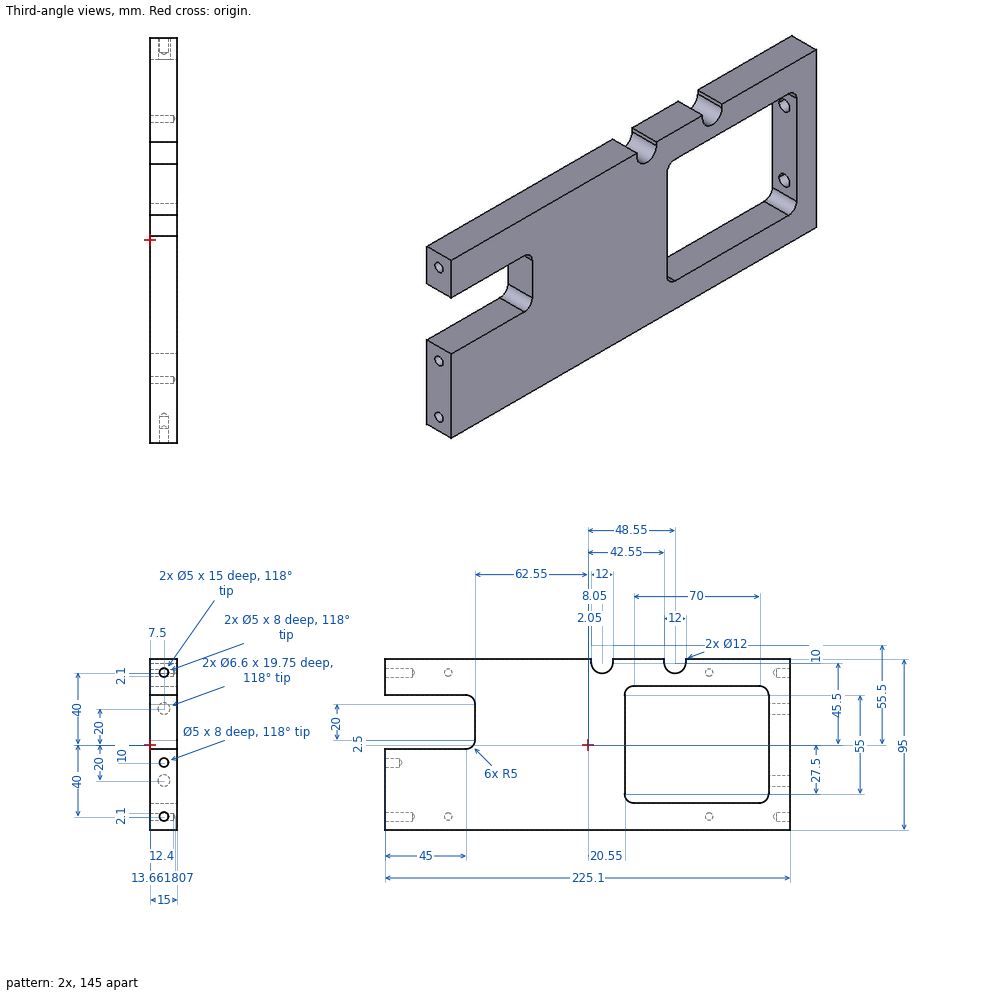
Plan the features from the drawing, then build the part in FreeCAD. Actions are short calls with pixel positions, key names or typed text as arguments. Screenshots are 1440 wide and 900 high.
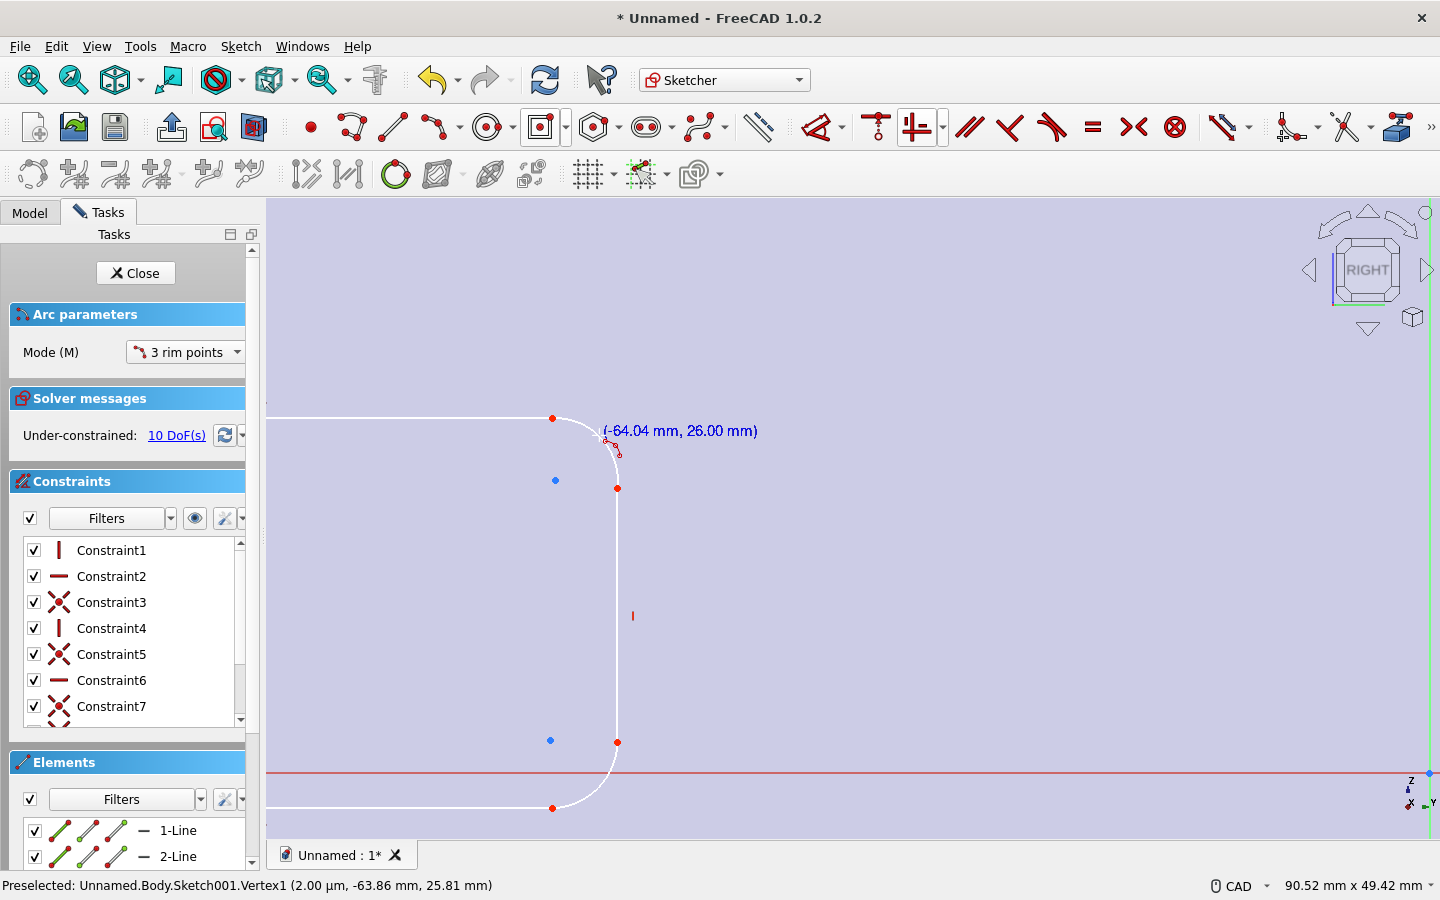
click(393, 128)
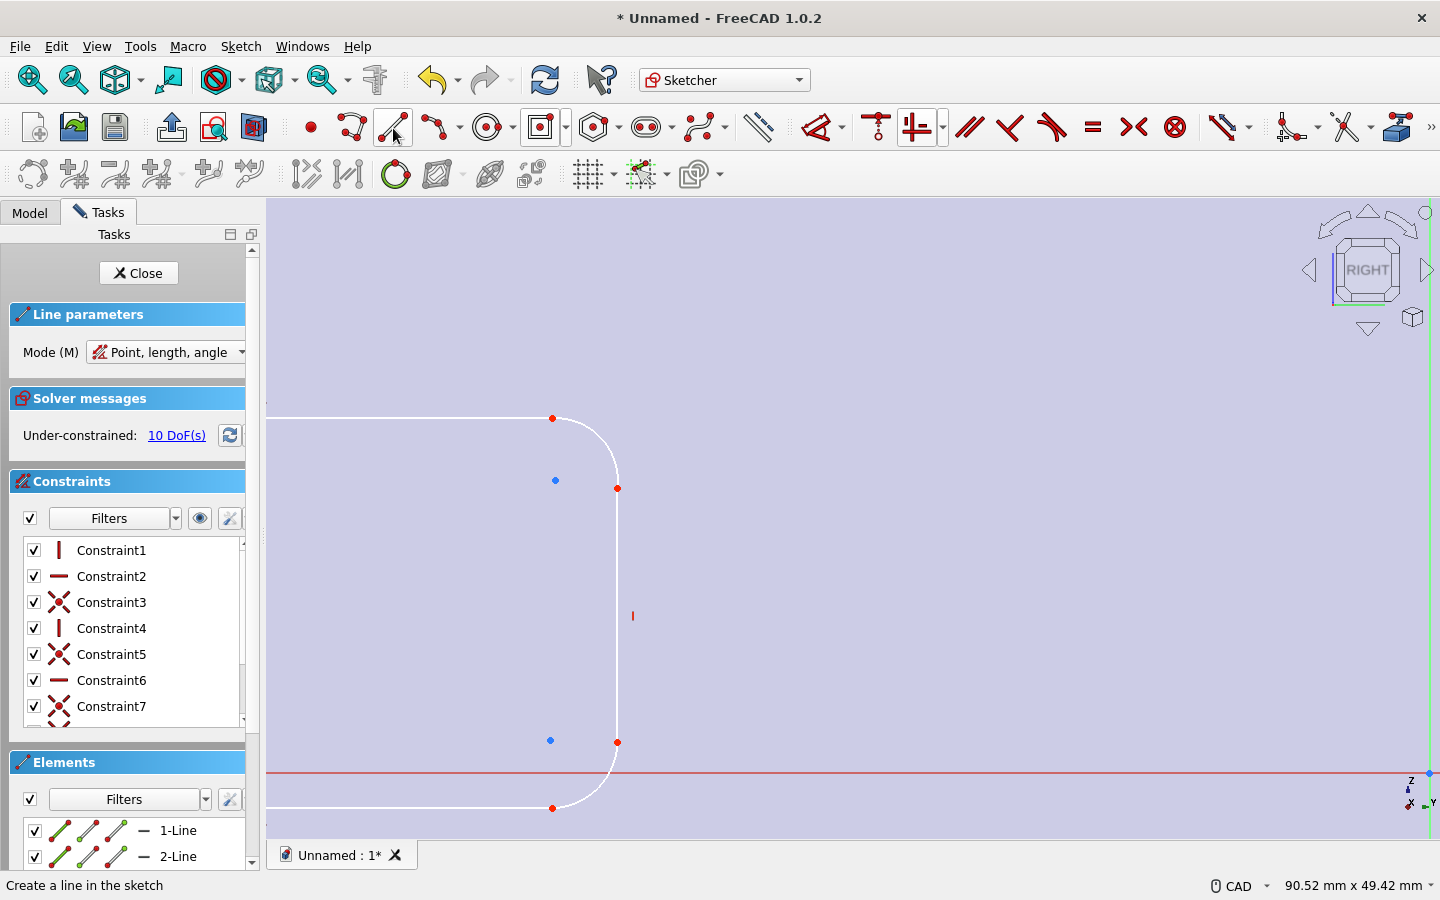
scroll(599, 435, down, 7)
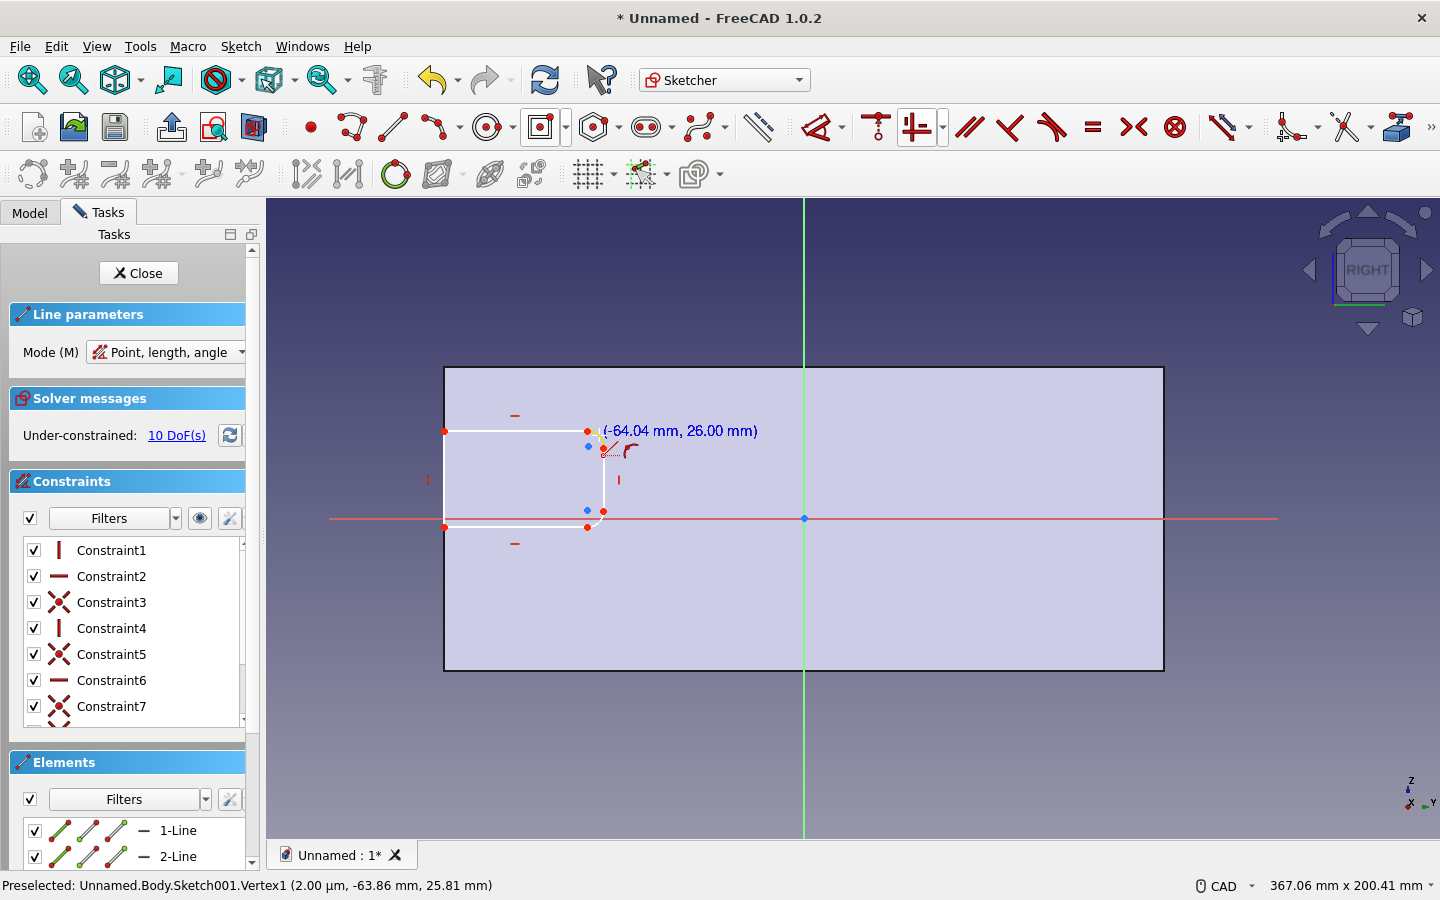
click(870, 607)
click(870, 431)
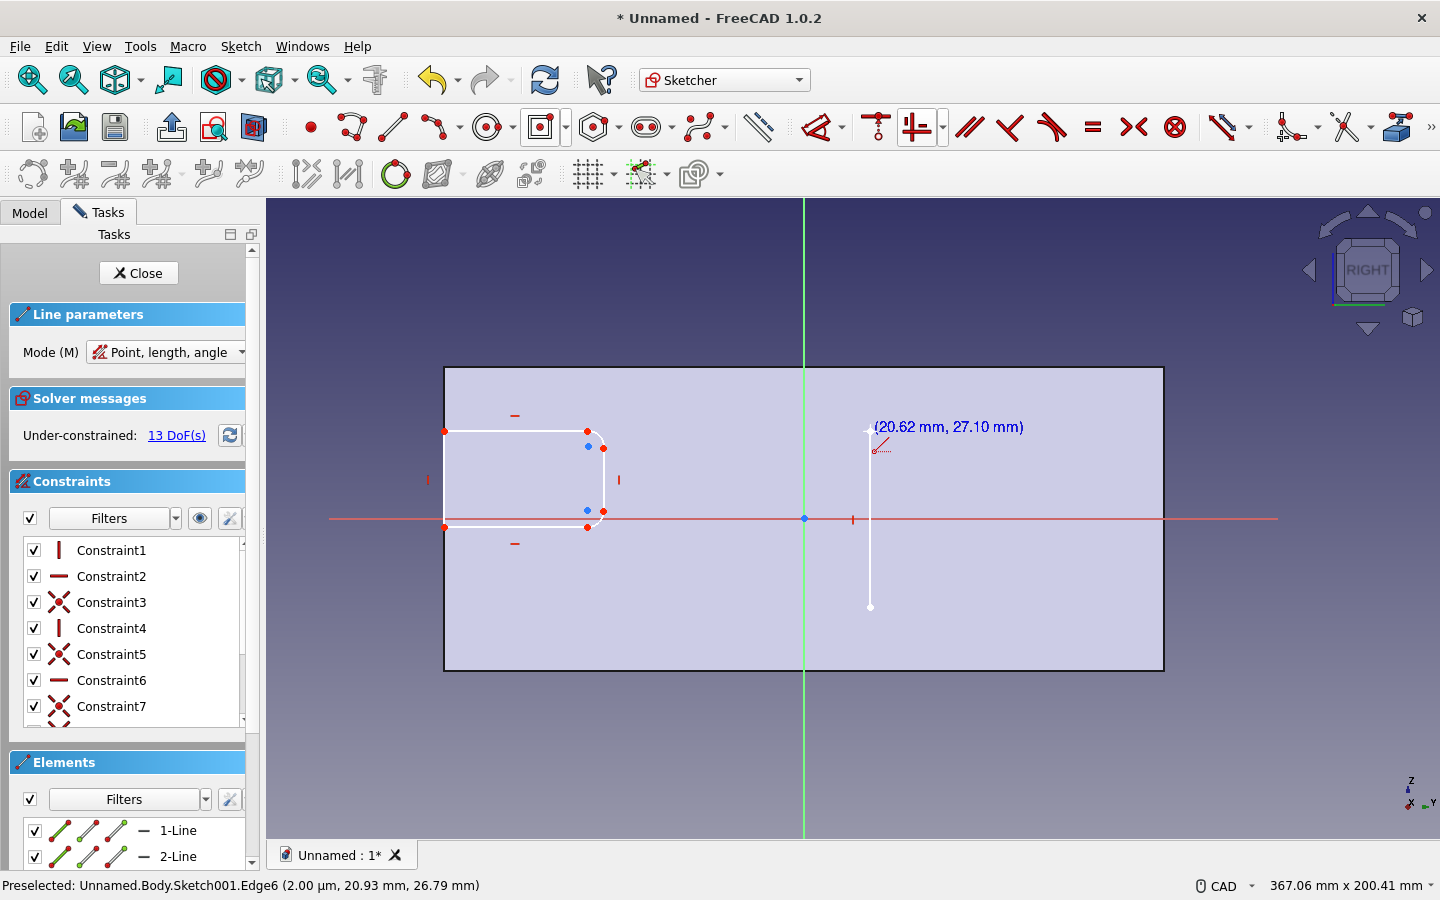
click(886, 415)
click(1110, 415)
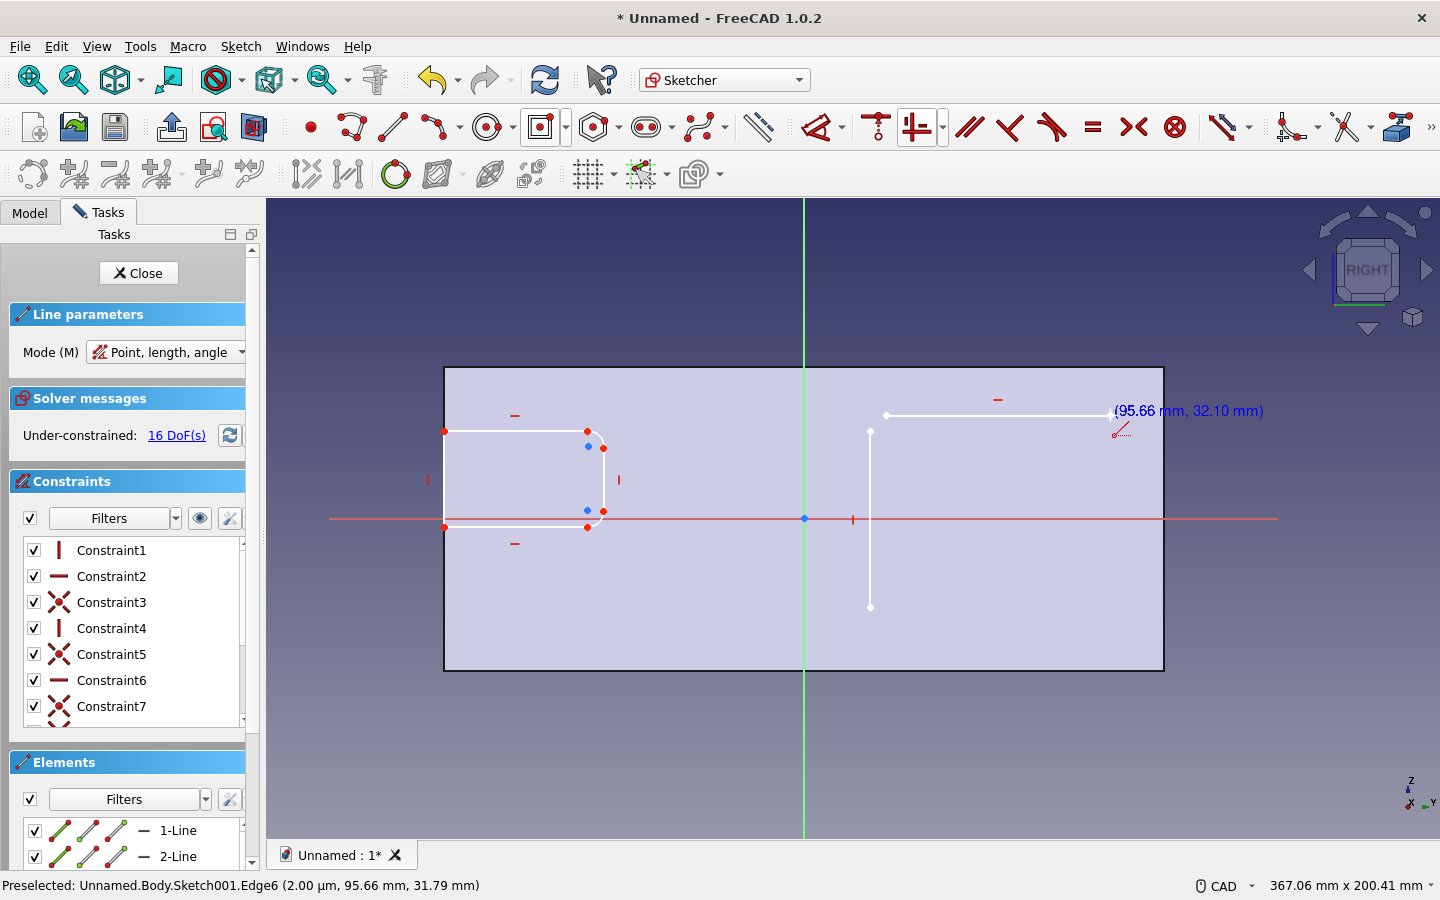
click(1126, 431)
click(1126, 607)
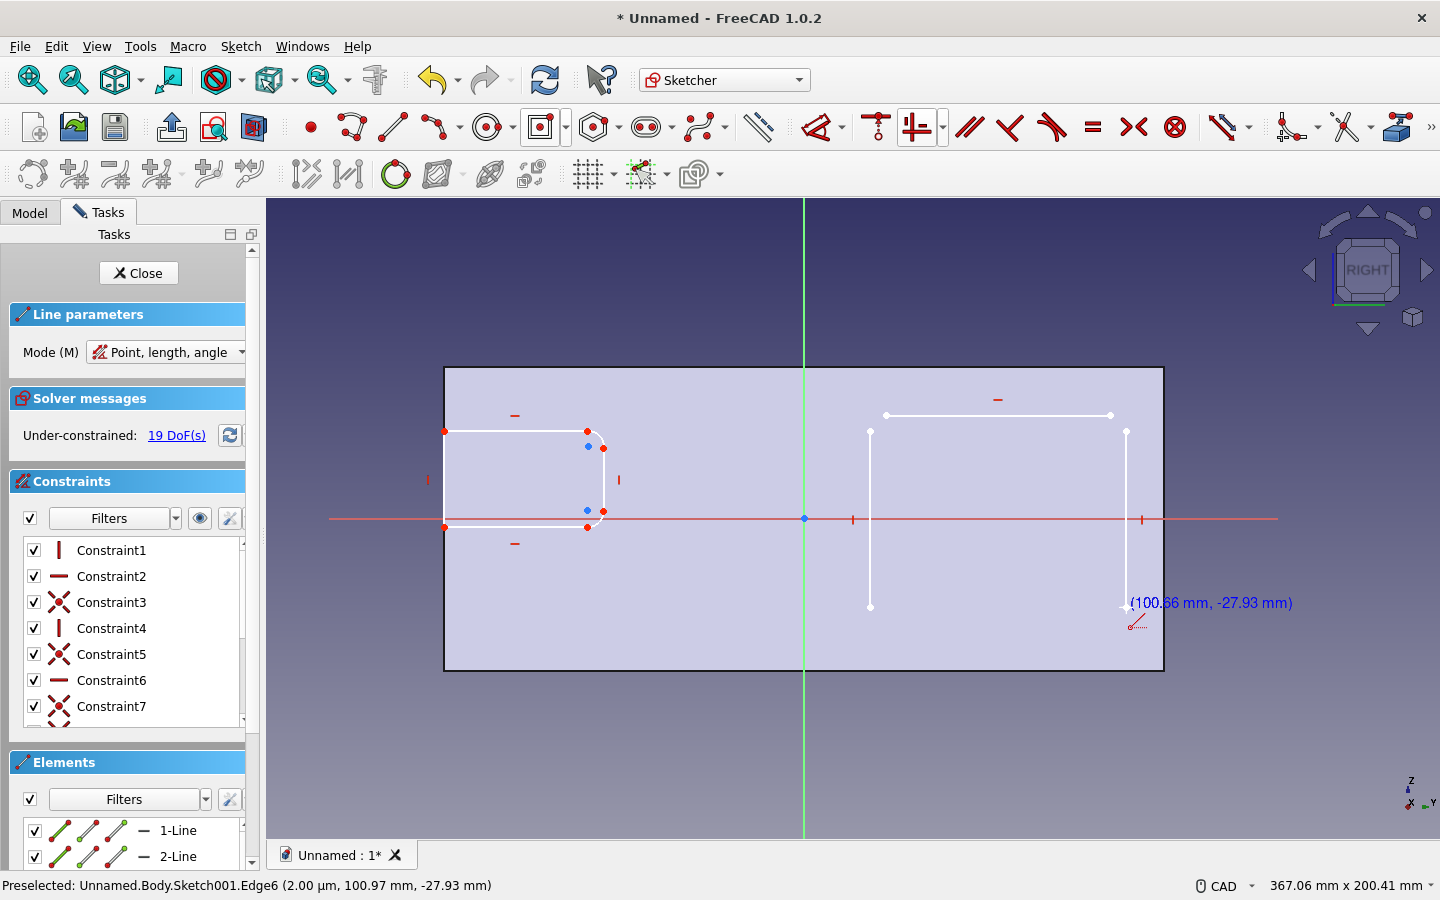
click(1110, 623)
click(886, 623)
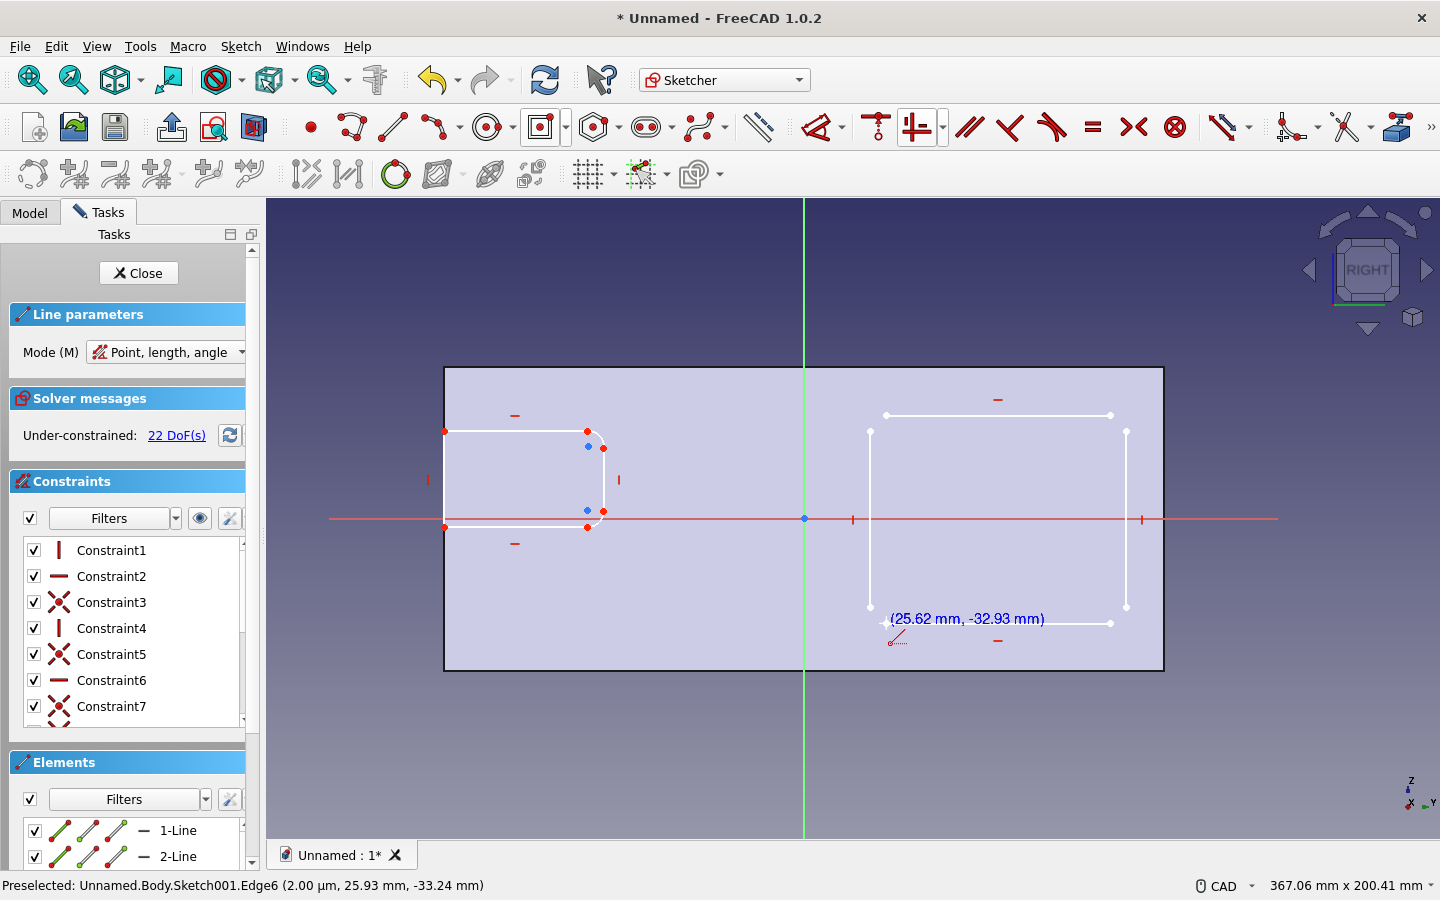
click(434, 128)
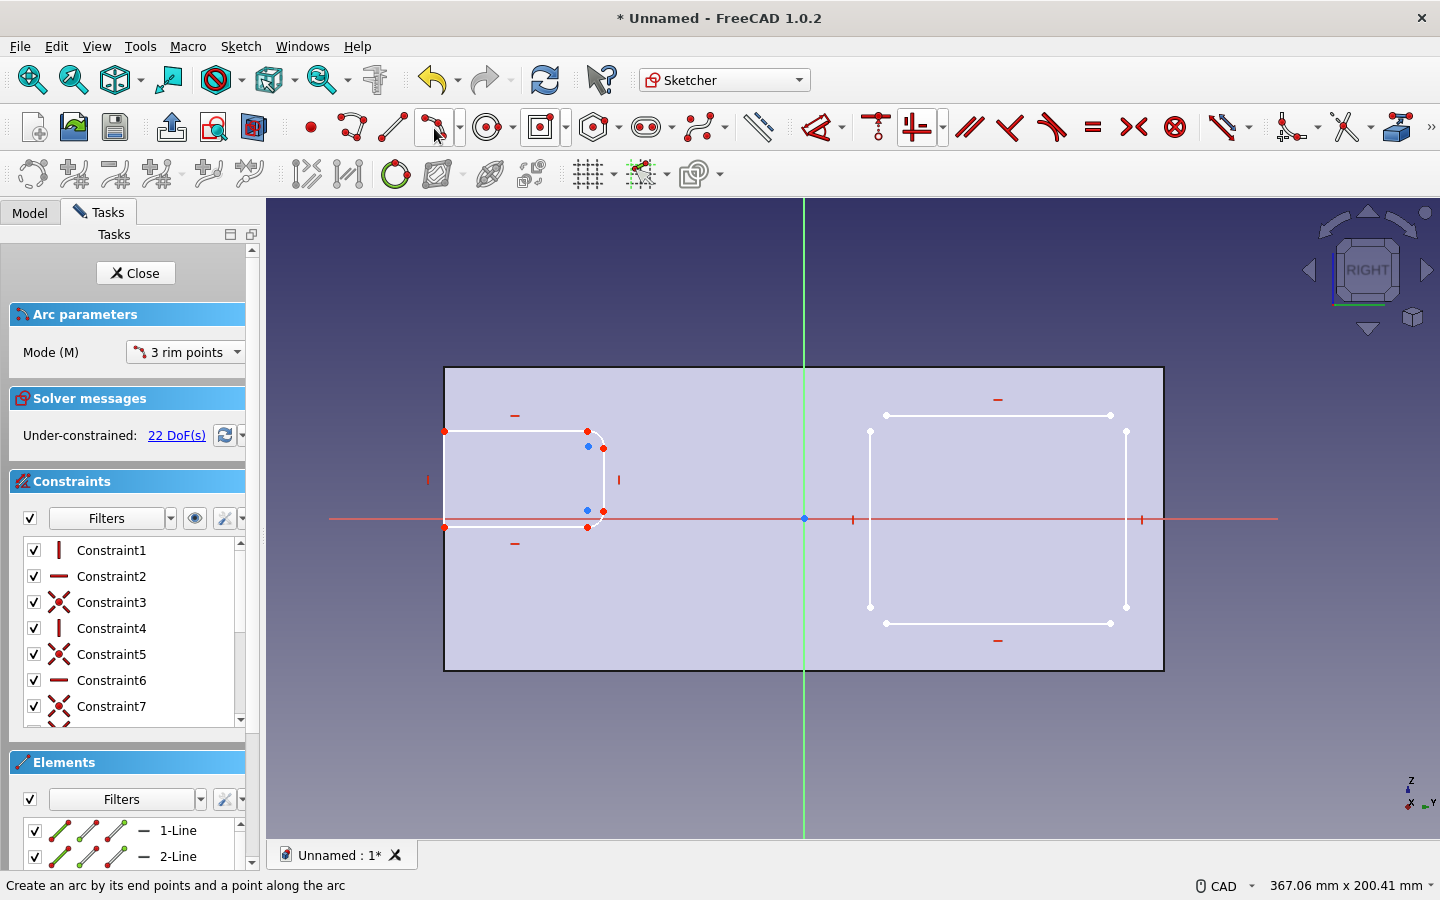
click(870, 432)
click(886, 416)